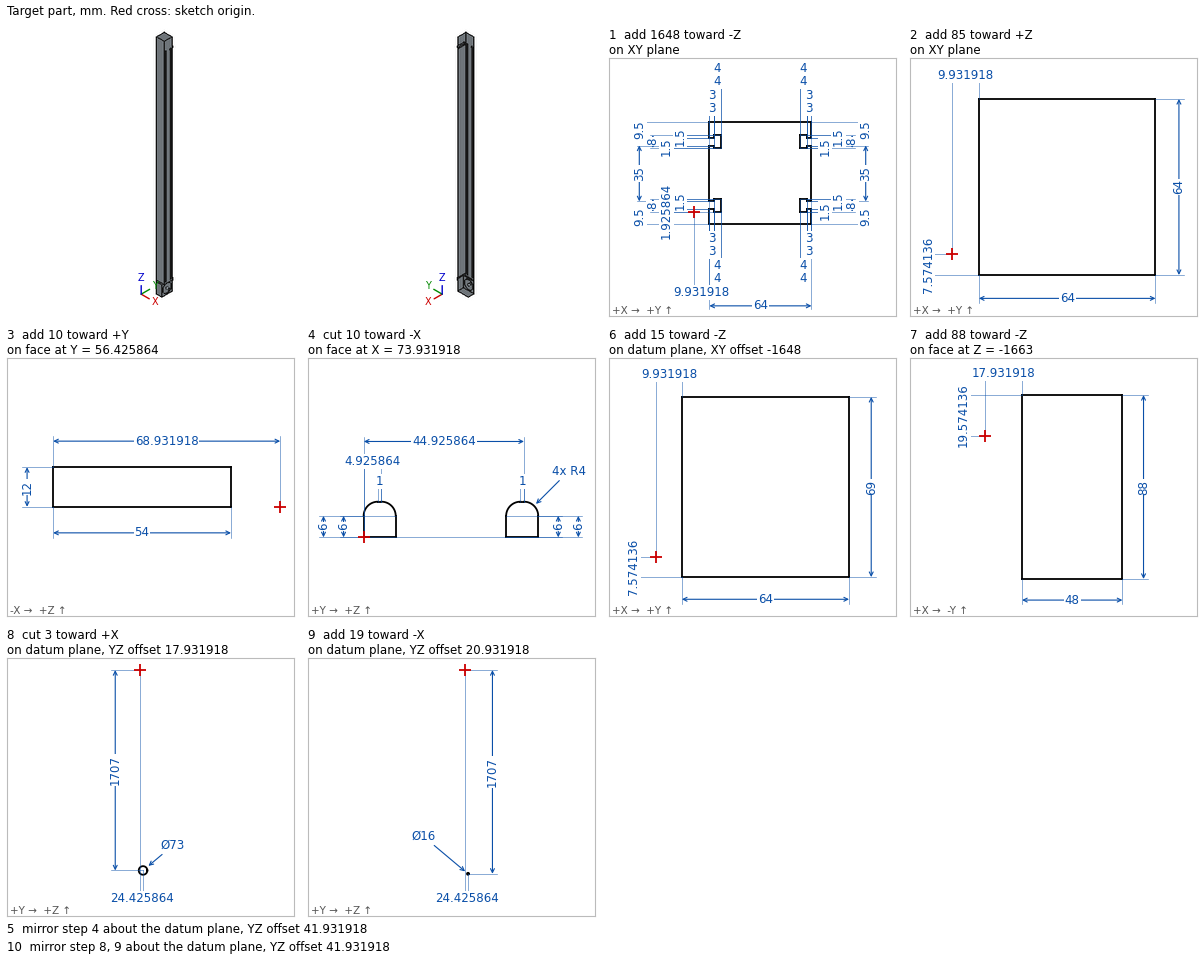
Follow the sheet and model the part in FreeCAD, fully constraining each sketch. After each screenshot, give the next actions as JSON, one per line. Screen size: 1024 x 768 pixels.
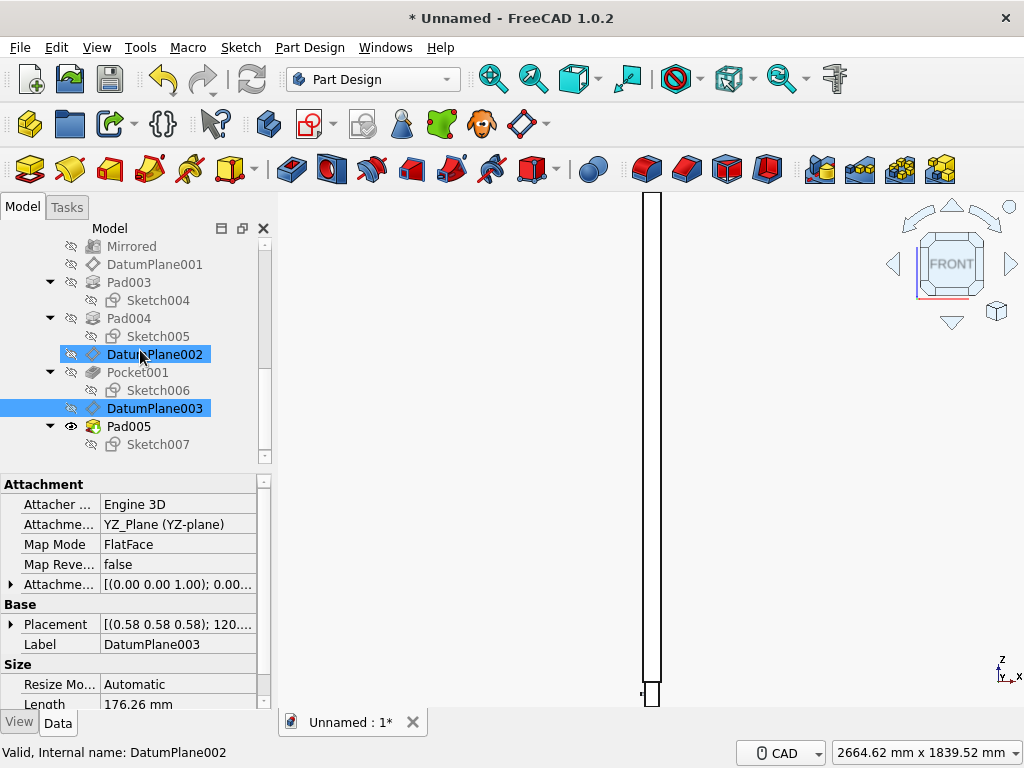
{"action": "scroll", "coordinate": [140, 350], "scroll_direction": "up", "scroll_amount": 15}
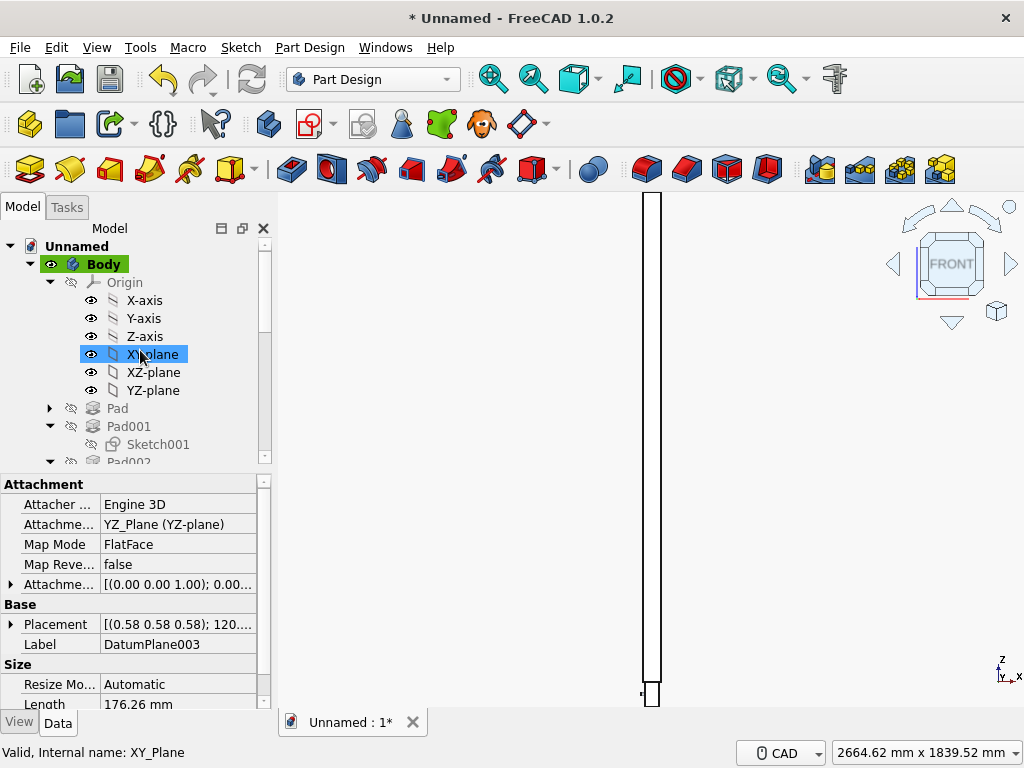
{"action": "left_click", "coordinate": [136, 390]}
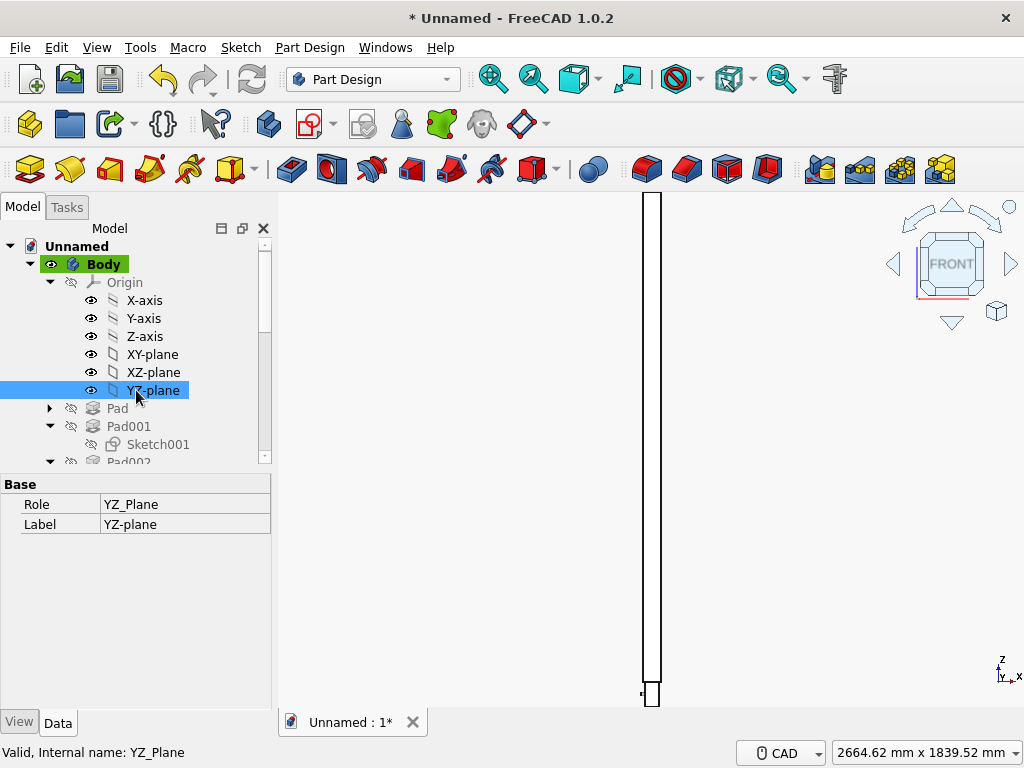
{"action": "left_click", "coordinate": [522, 124]}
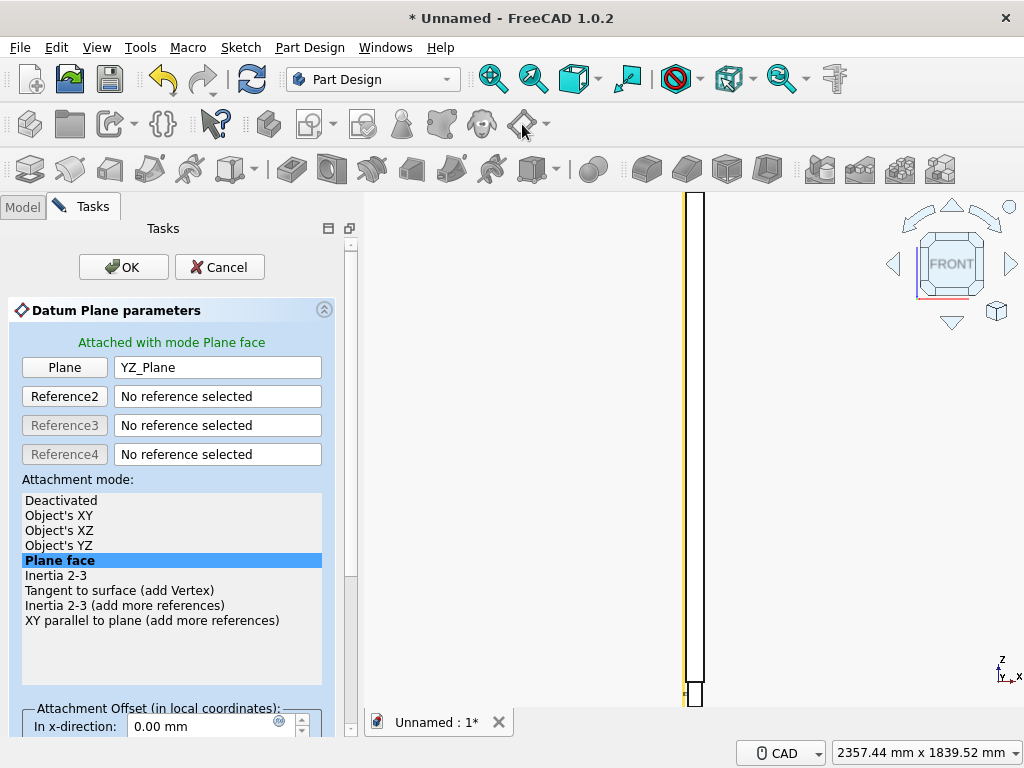
{"action": "scroll", "coordinate": [351, 487], "scroll_direction": "down", "scroll_amount": 3}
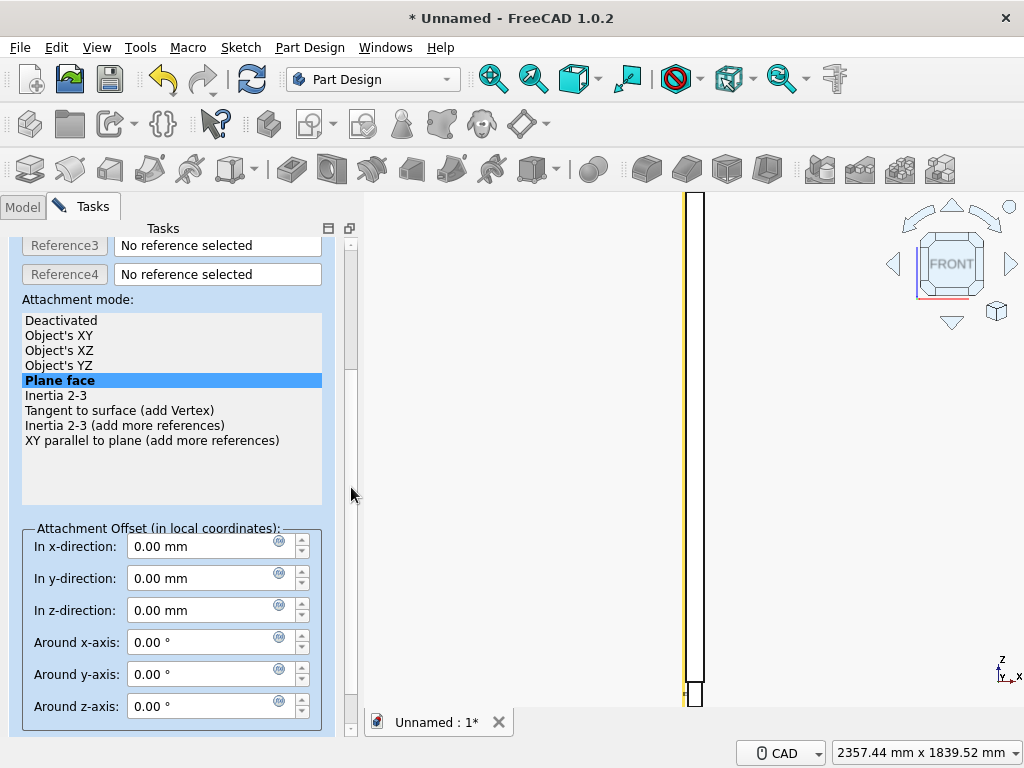
{"action": "triple_click", "coordinate": [210, 610]}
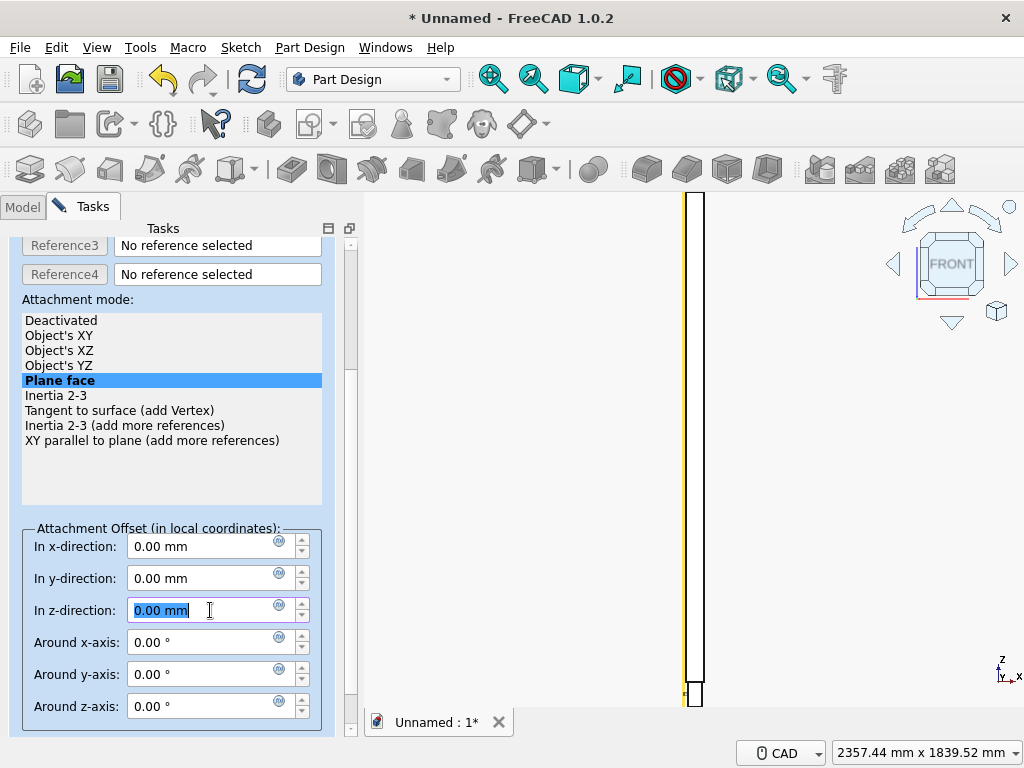
{"action": "type", "text": "41.931918"}
{"action": "key", "text": "Tab"}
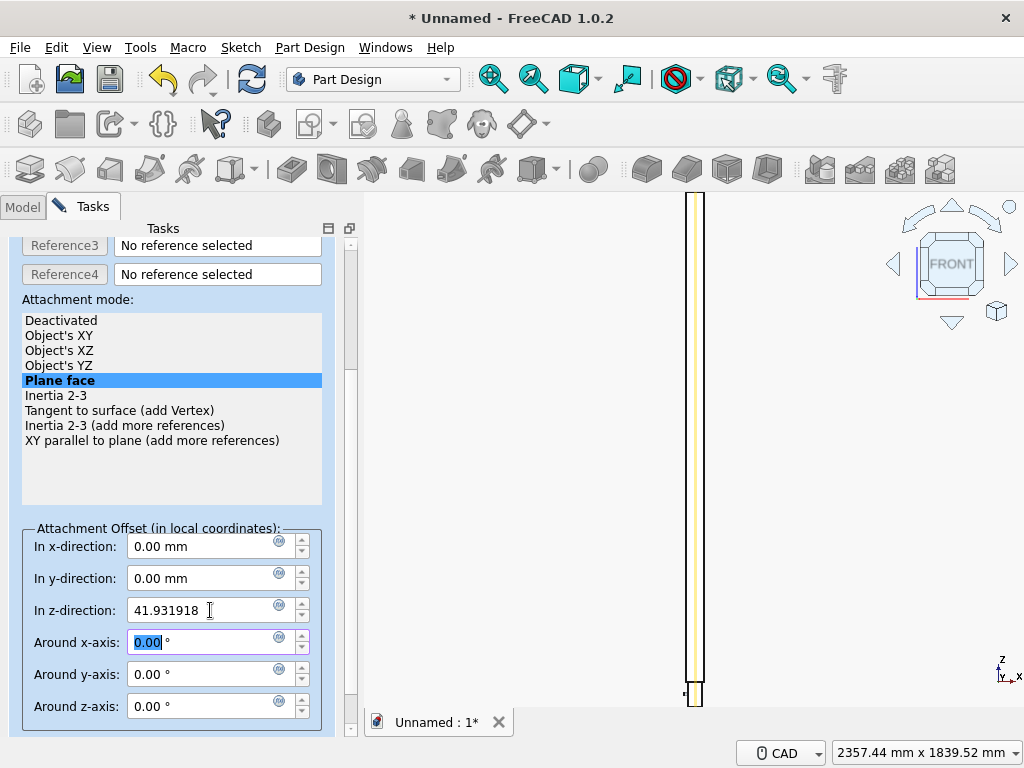
{"action": "scroll", "coordinate": [351, 487], "scroll_direction": "up", "scroll_amount": 4}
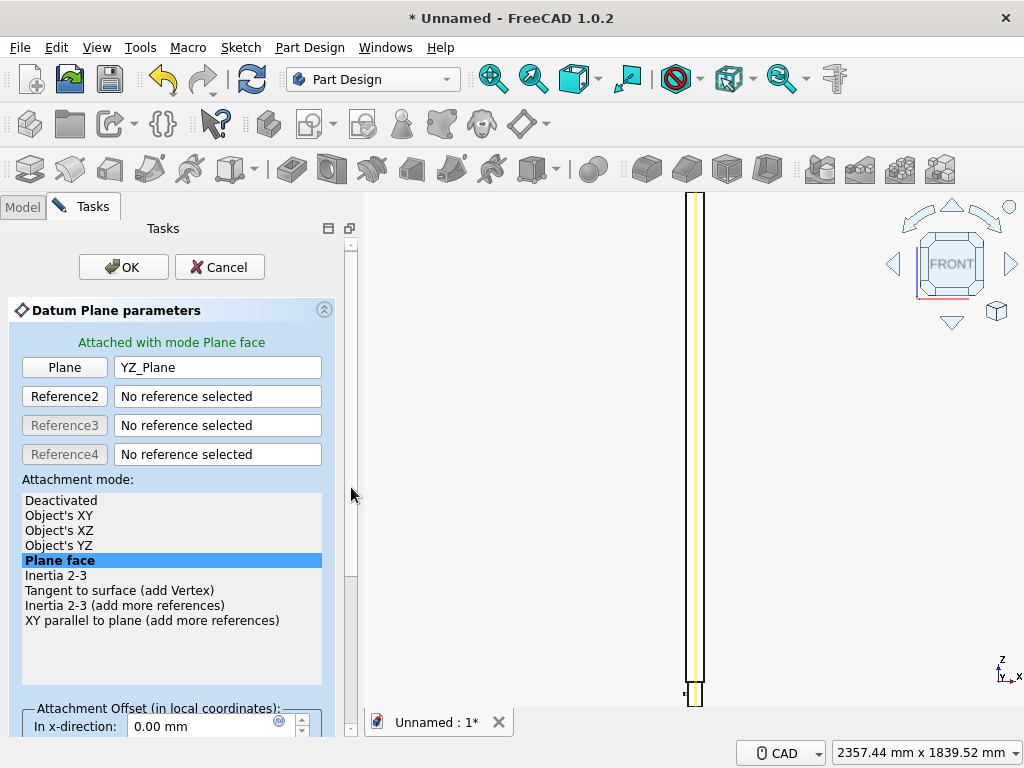
{"action": "left_click", "coordinate": [124, 267]}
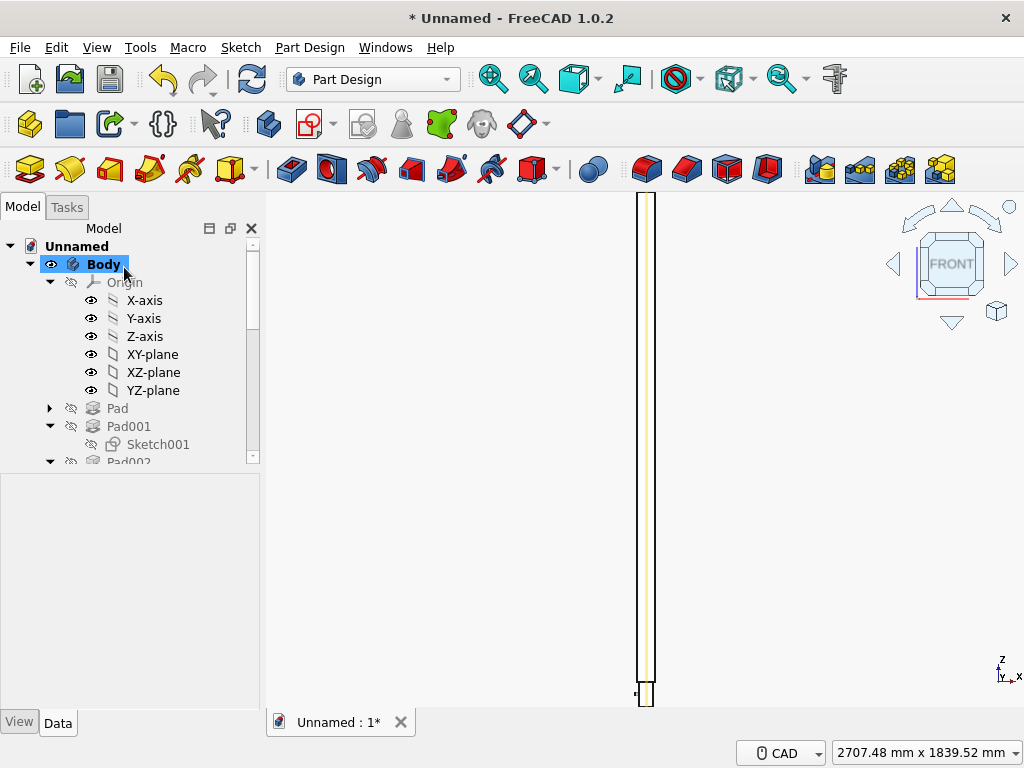
{"action": "scroll", "coordinate": [100, 350], "scroll_direction": "down", "scroll_amount": 3}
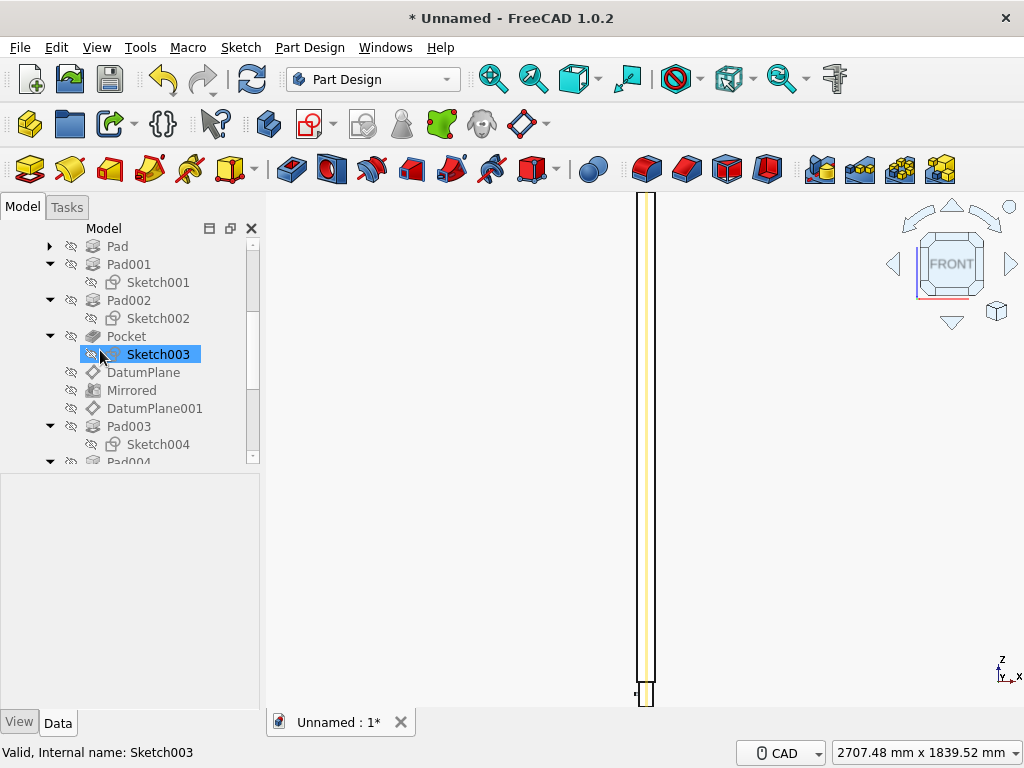
{"action": "scroll", "coordinate": [140, 350], "scroll_direction": "up", "scroll_amount": 15}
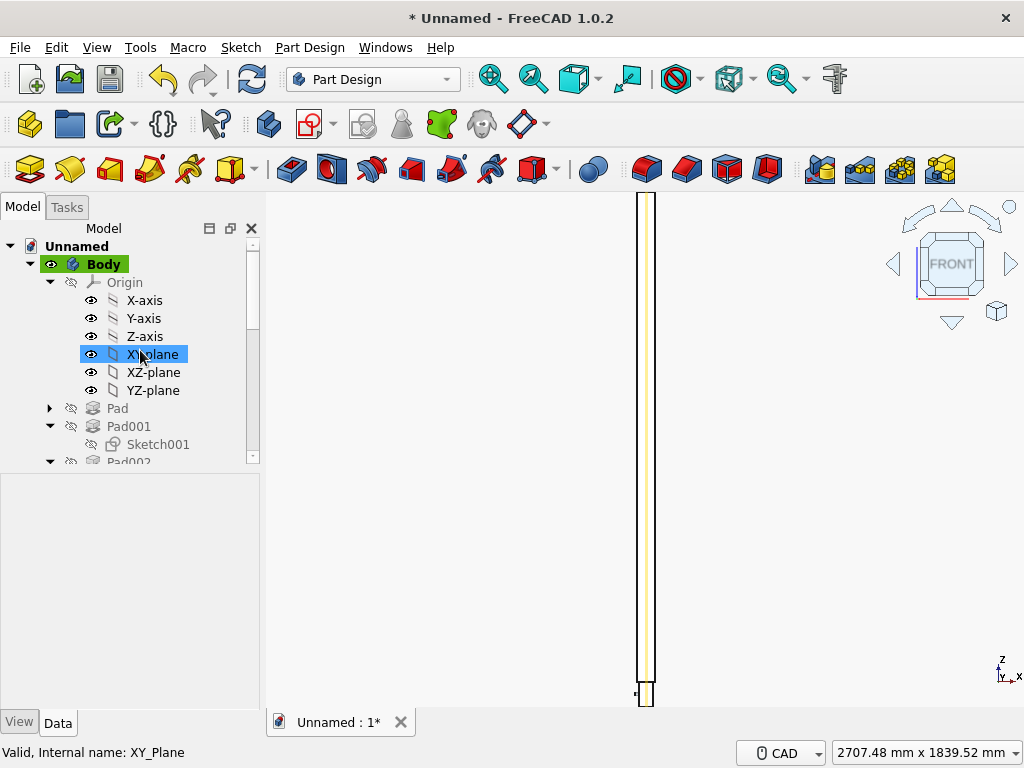
{"action": "scroll", "coordinate": [100, 350], "scroll_direction": "down", "scroll_amount": 6}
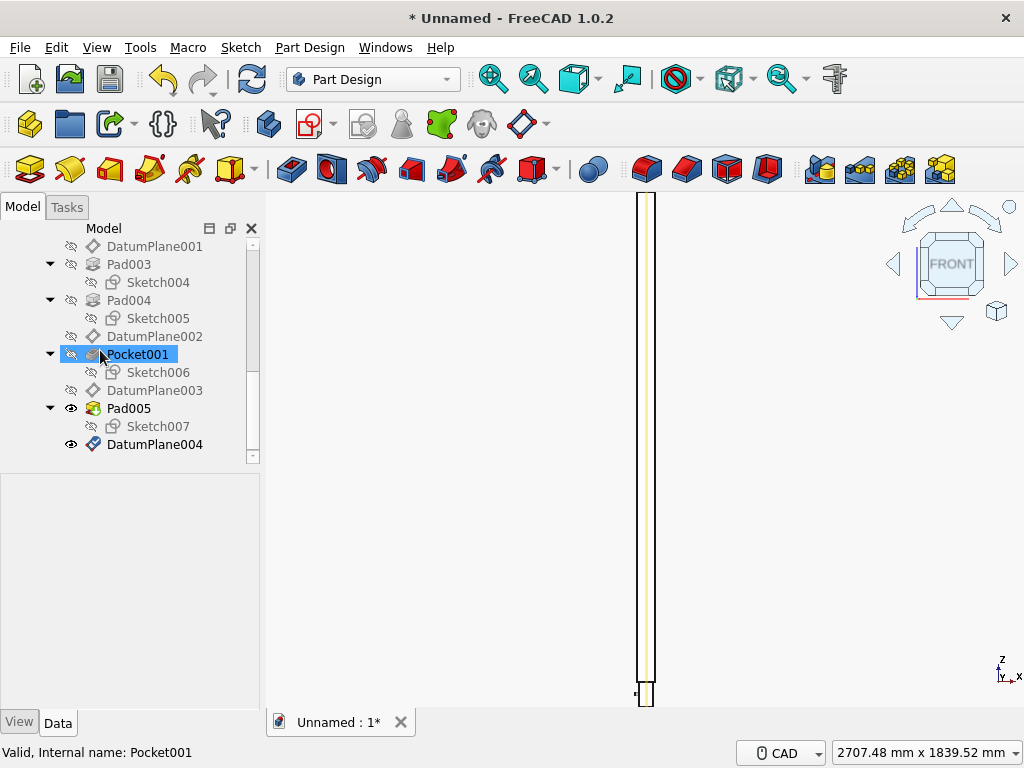
{"action": "left_click", "coordinate": [116, 354]}